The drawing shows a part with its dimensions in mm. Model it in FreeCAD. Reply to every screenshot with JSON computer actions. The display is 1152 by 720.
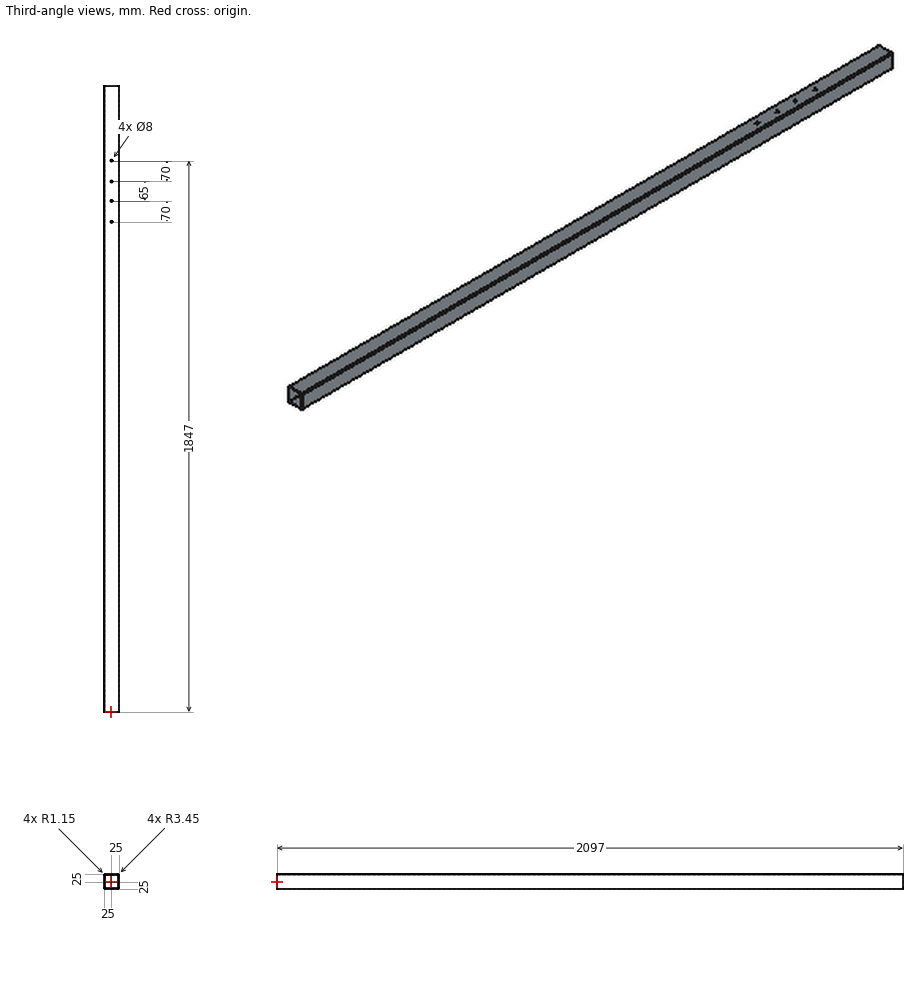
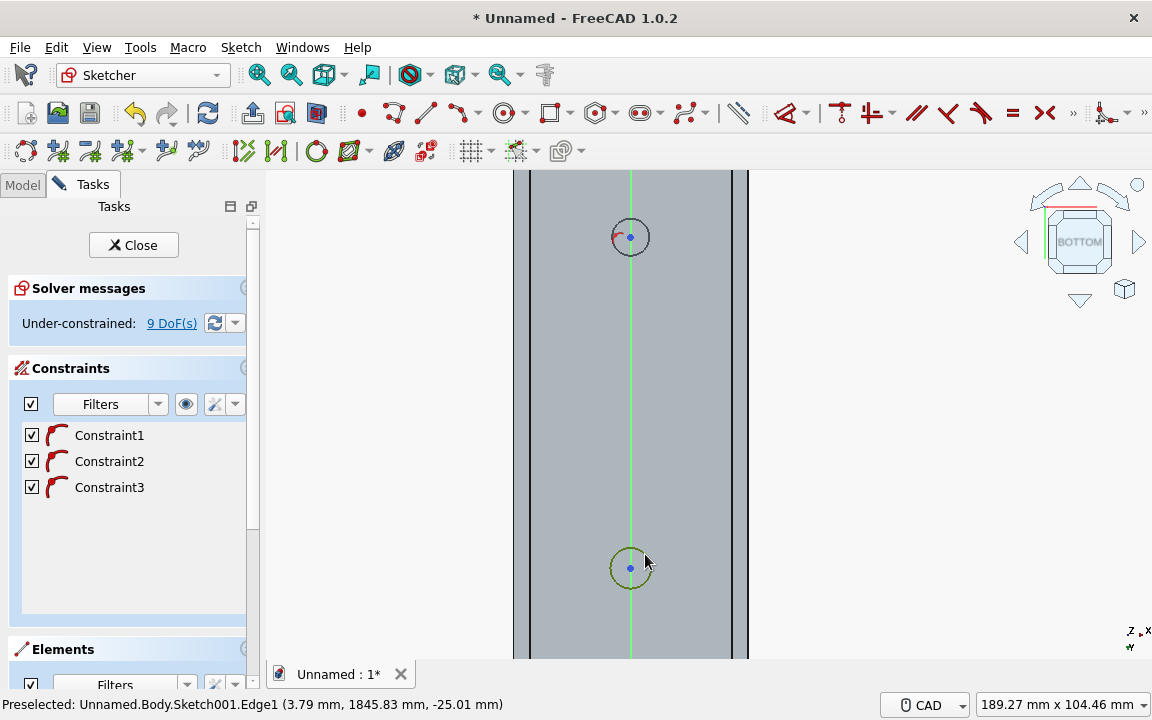
{"action": "left_click", "coordinate": [644, 224]}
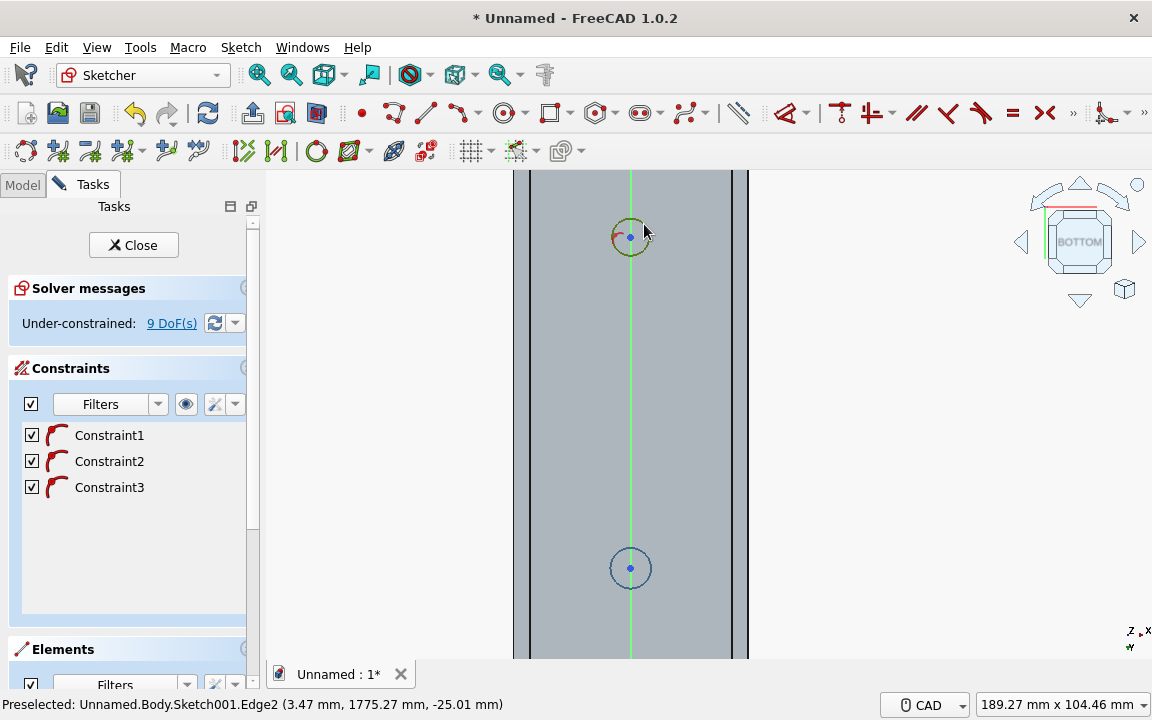
{"action": "scroll", "coordinate": [645, 557], "scroll_direction": "down", "scroll_amount": 6}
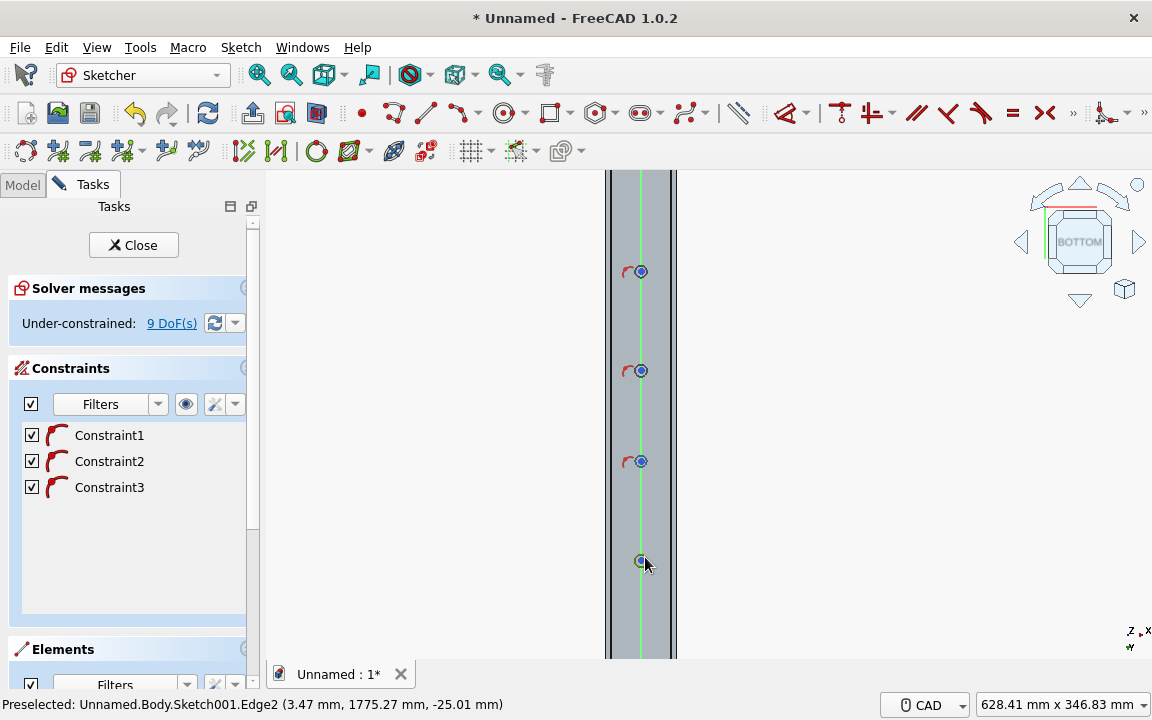
{"action": "scroll", "coordinate": [645, 366], "scroll_direction": "up", "scroll_amount": 6}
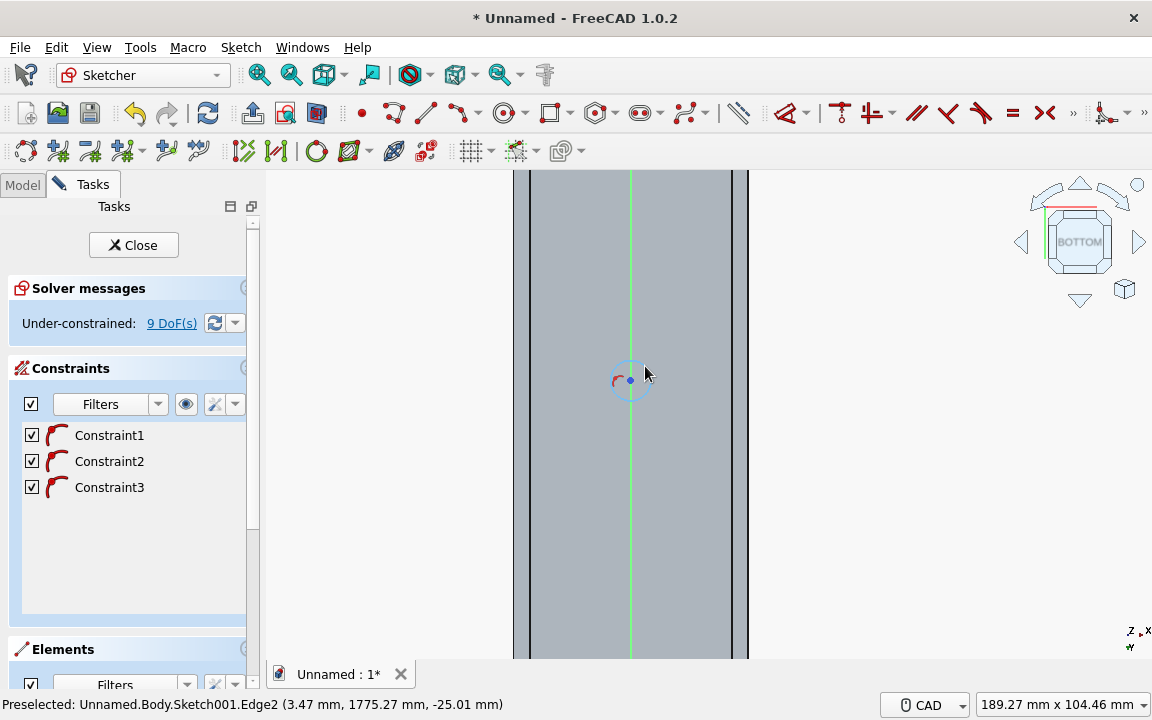
{"action": "left_click", "coordinate": [645, 366]}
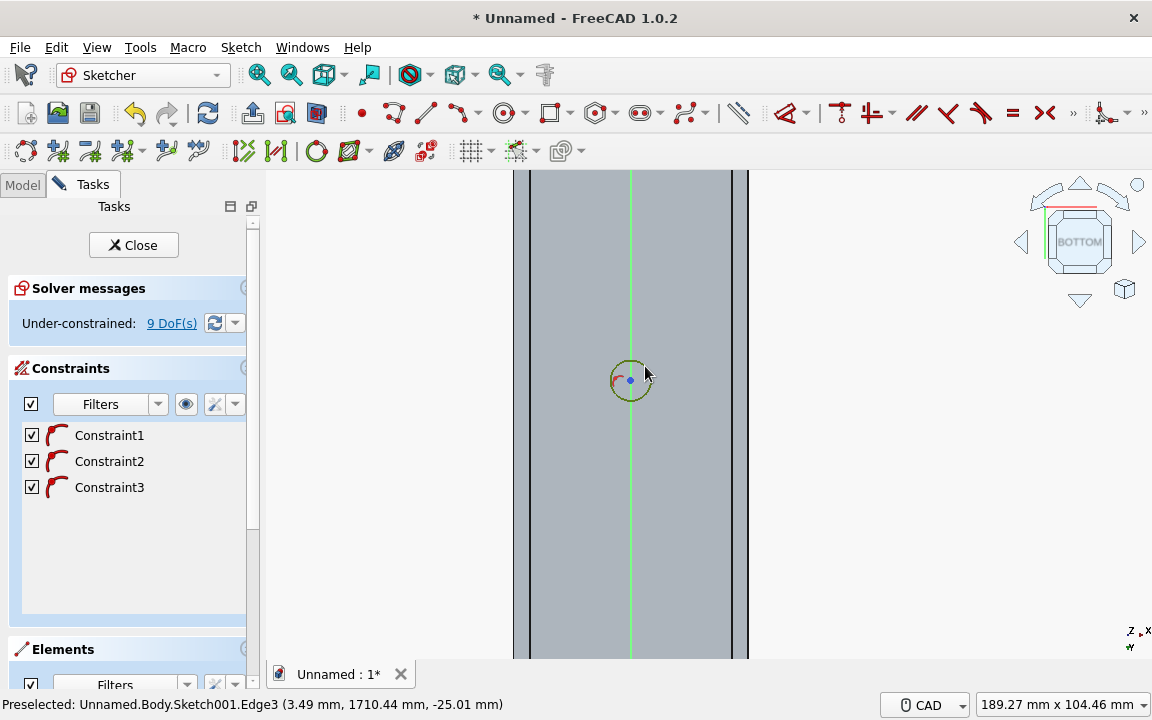
{"action": "scroll", "coordinate": [645, 365], "scroll_direction": "down", "scroll_amount": 6}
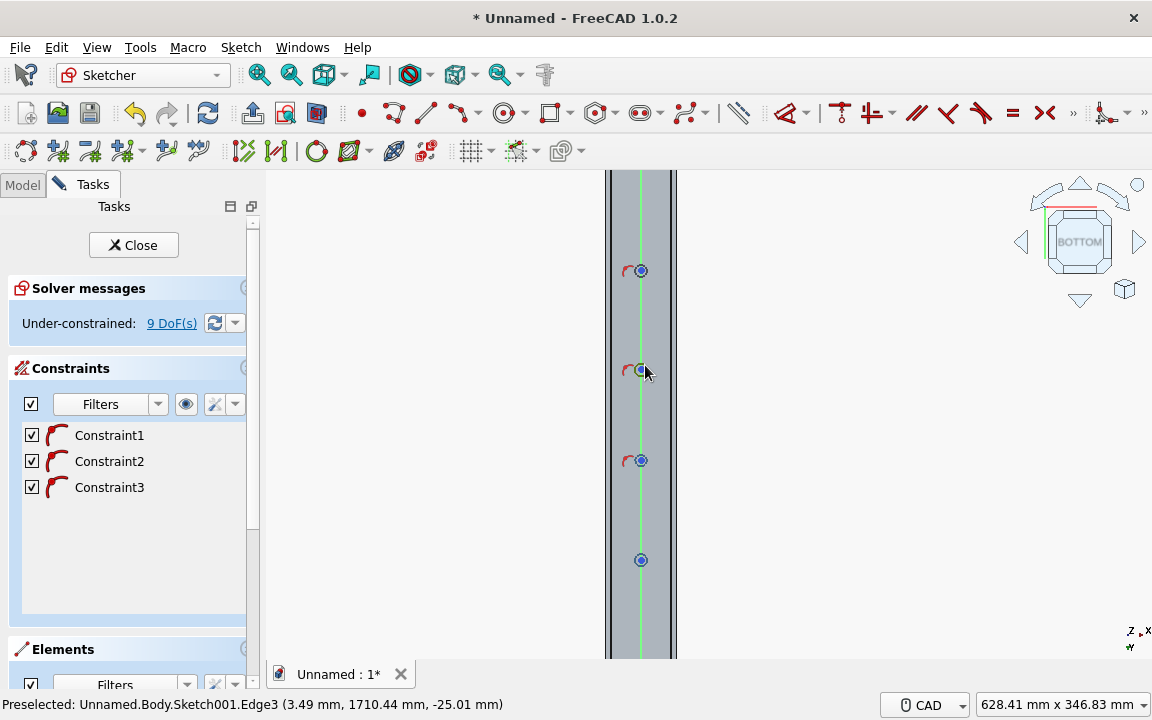
{"action": "scroll", "coordinate": [645, 267], "scroll_direction": "up", "scroll_amount": 7}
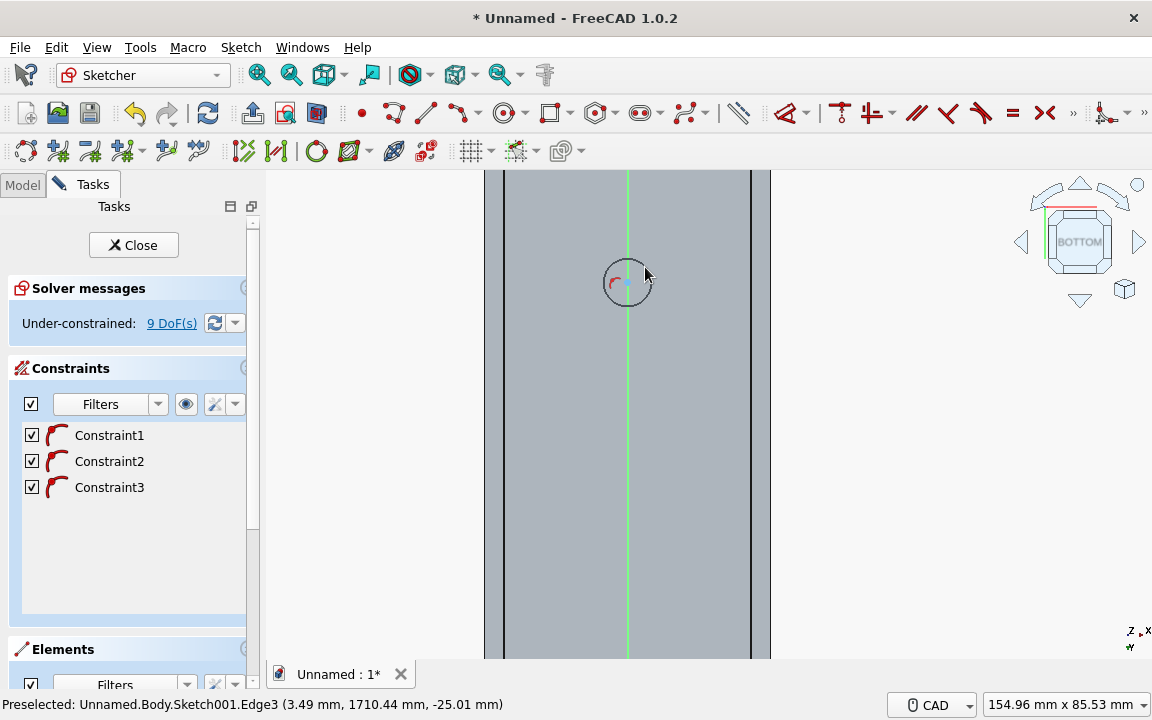
{"action": "left_click", "coordinate": [644, 266]}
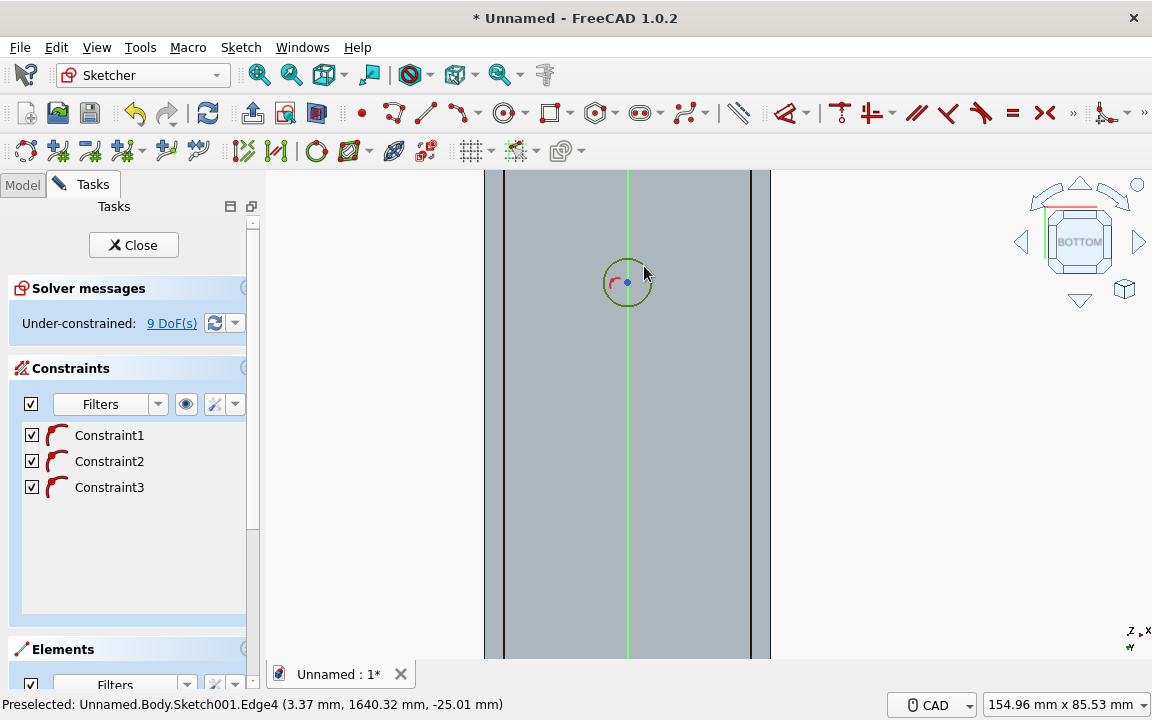
{"action": "left_click", "coordinate": [1014, 114]}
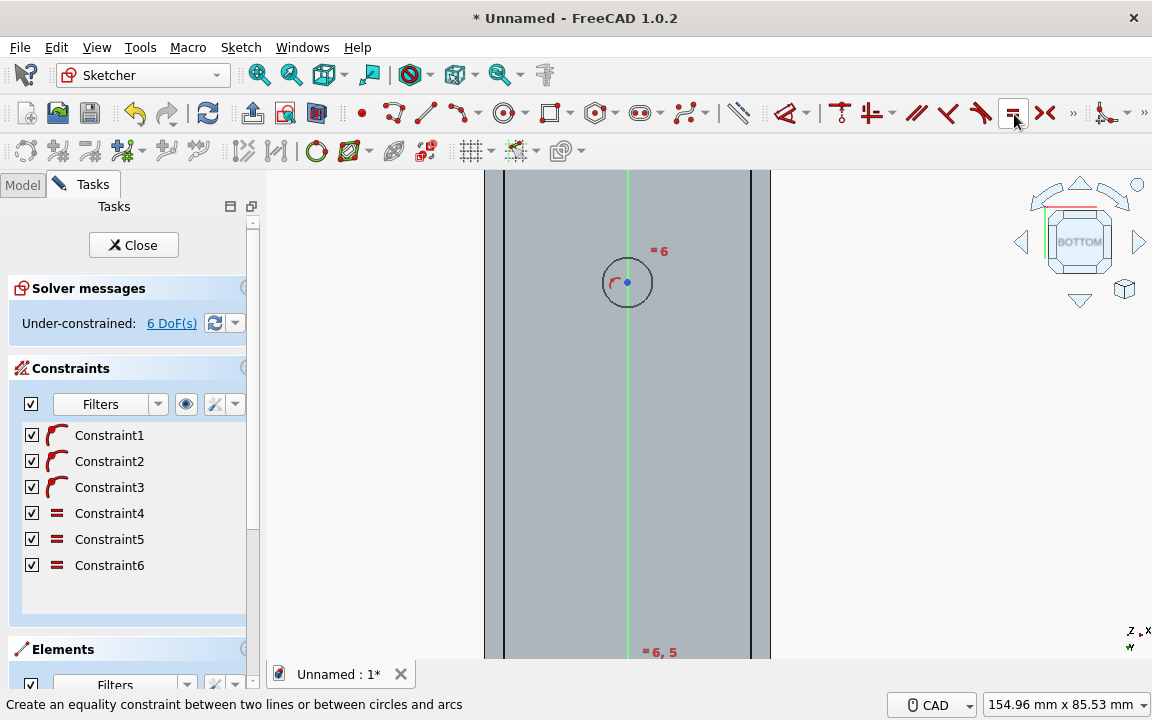
{"action": "scroll", "coordinate": [645, 267], "scroll_direction": "down", "scroll_amount": 7}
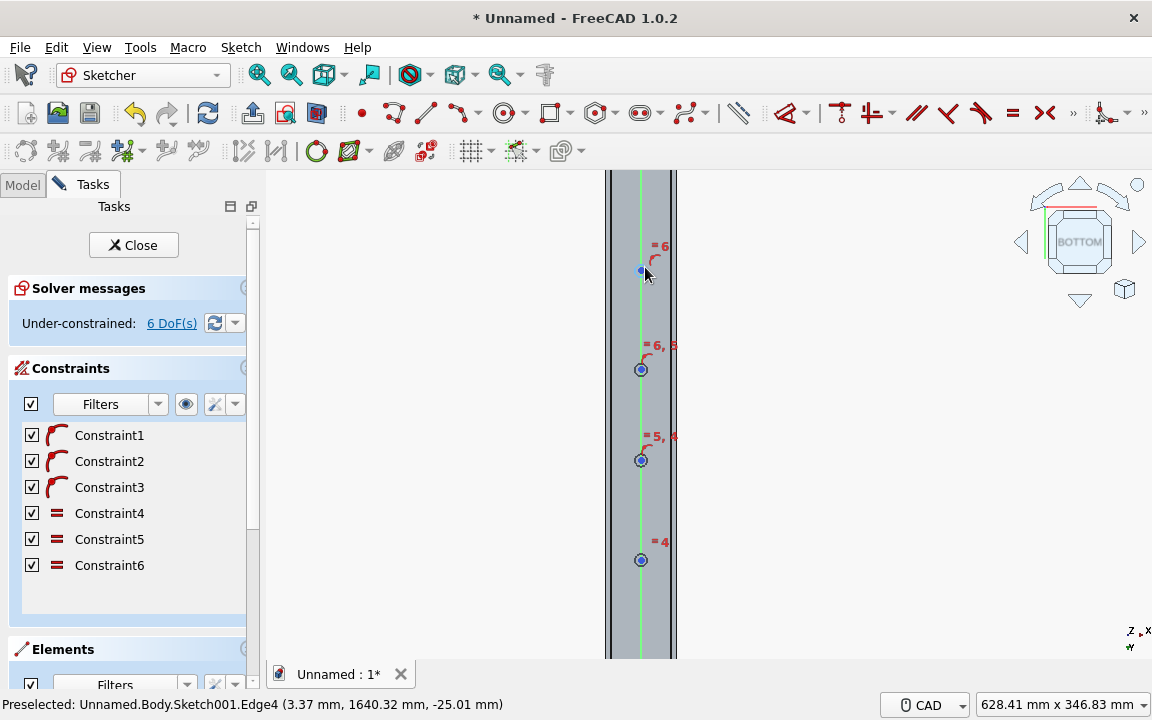
{"action": "left_click", "coordinate": [641, 560]}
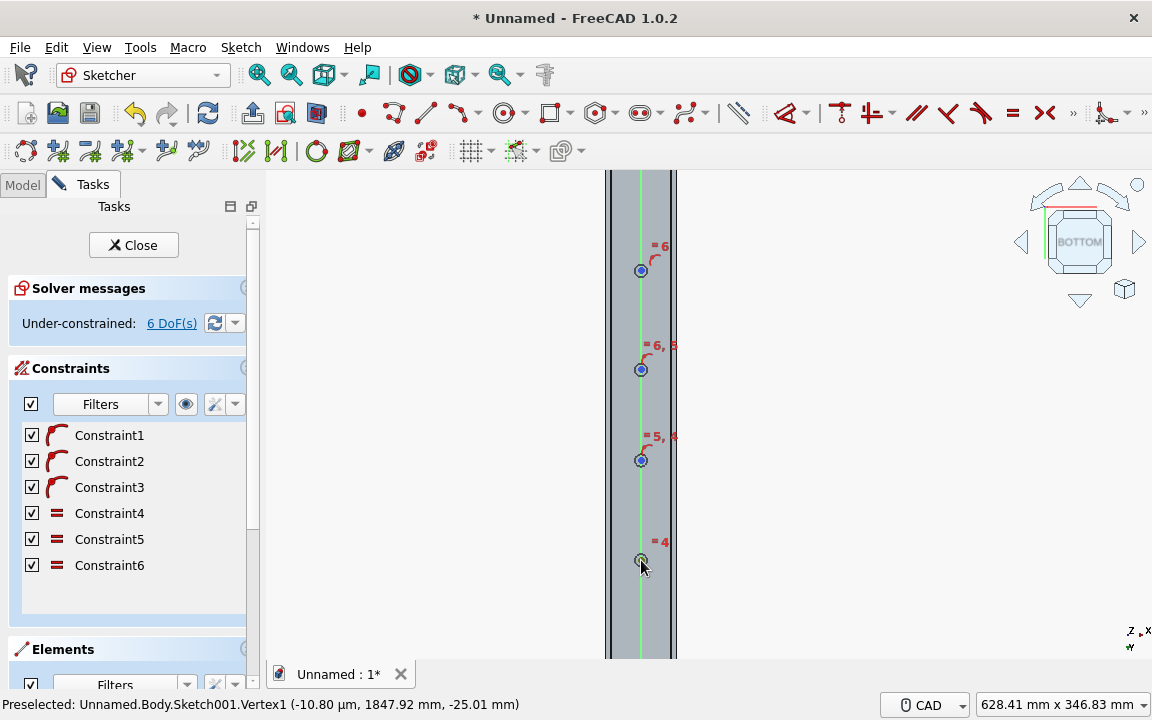
{"action": "left_click", "coordinate": [641, 600]}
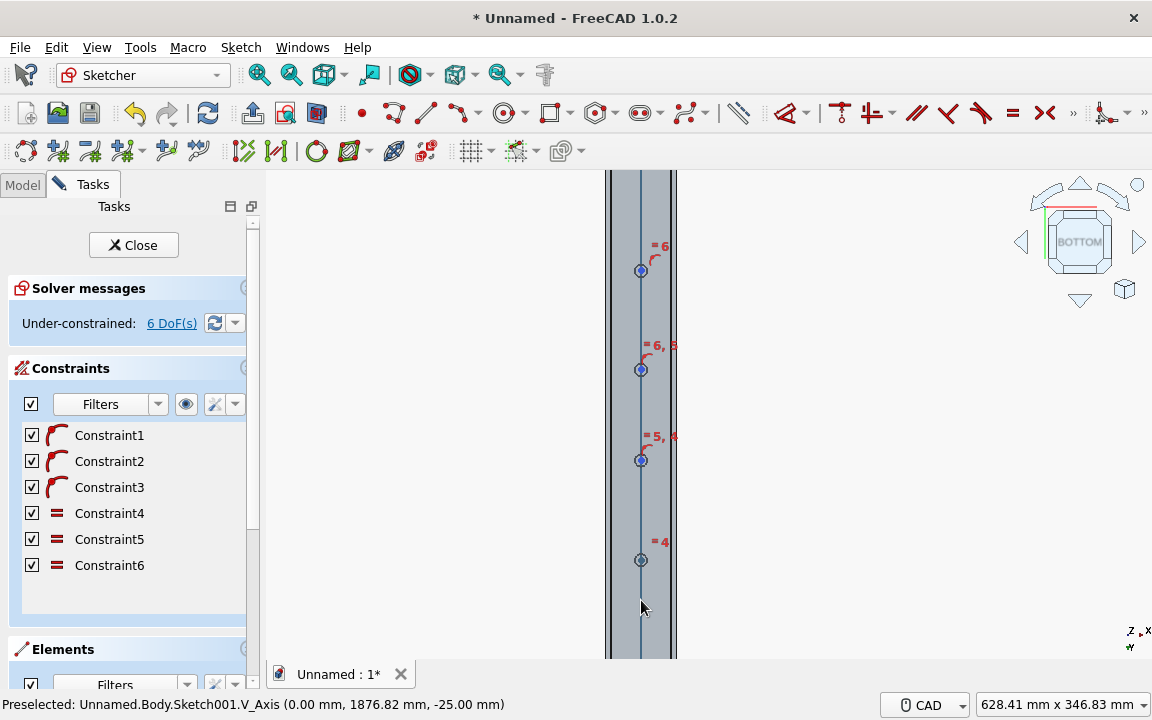
{"action": "left_click", "coordinate": [840, 114]}